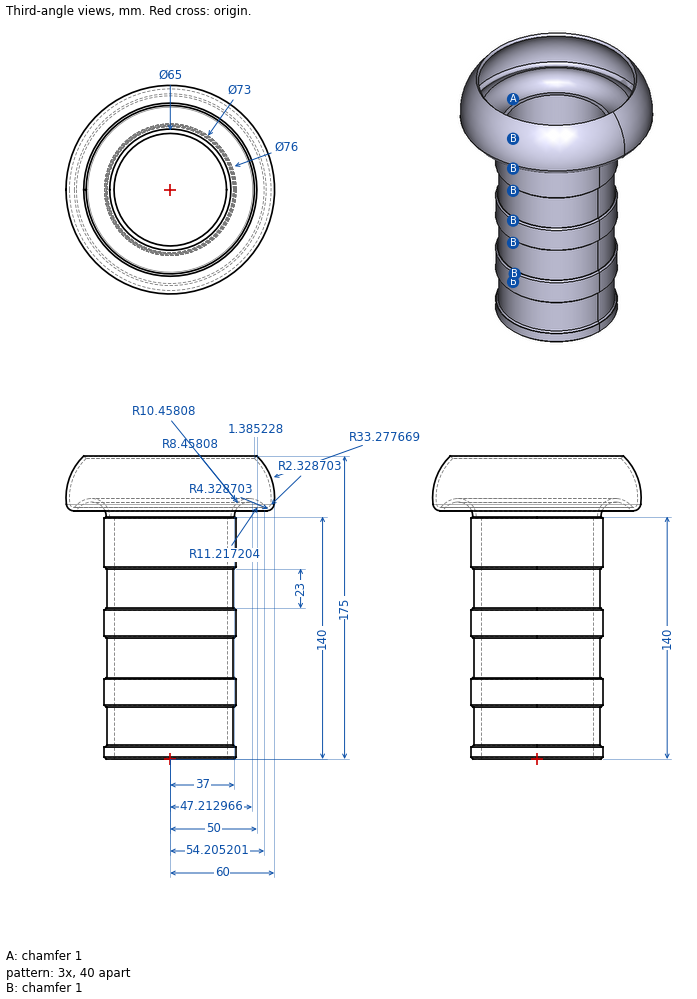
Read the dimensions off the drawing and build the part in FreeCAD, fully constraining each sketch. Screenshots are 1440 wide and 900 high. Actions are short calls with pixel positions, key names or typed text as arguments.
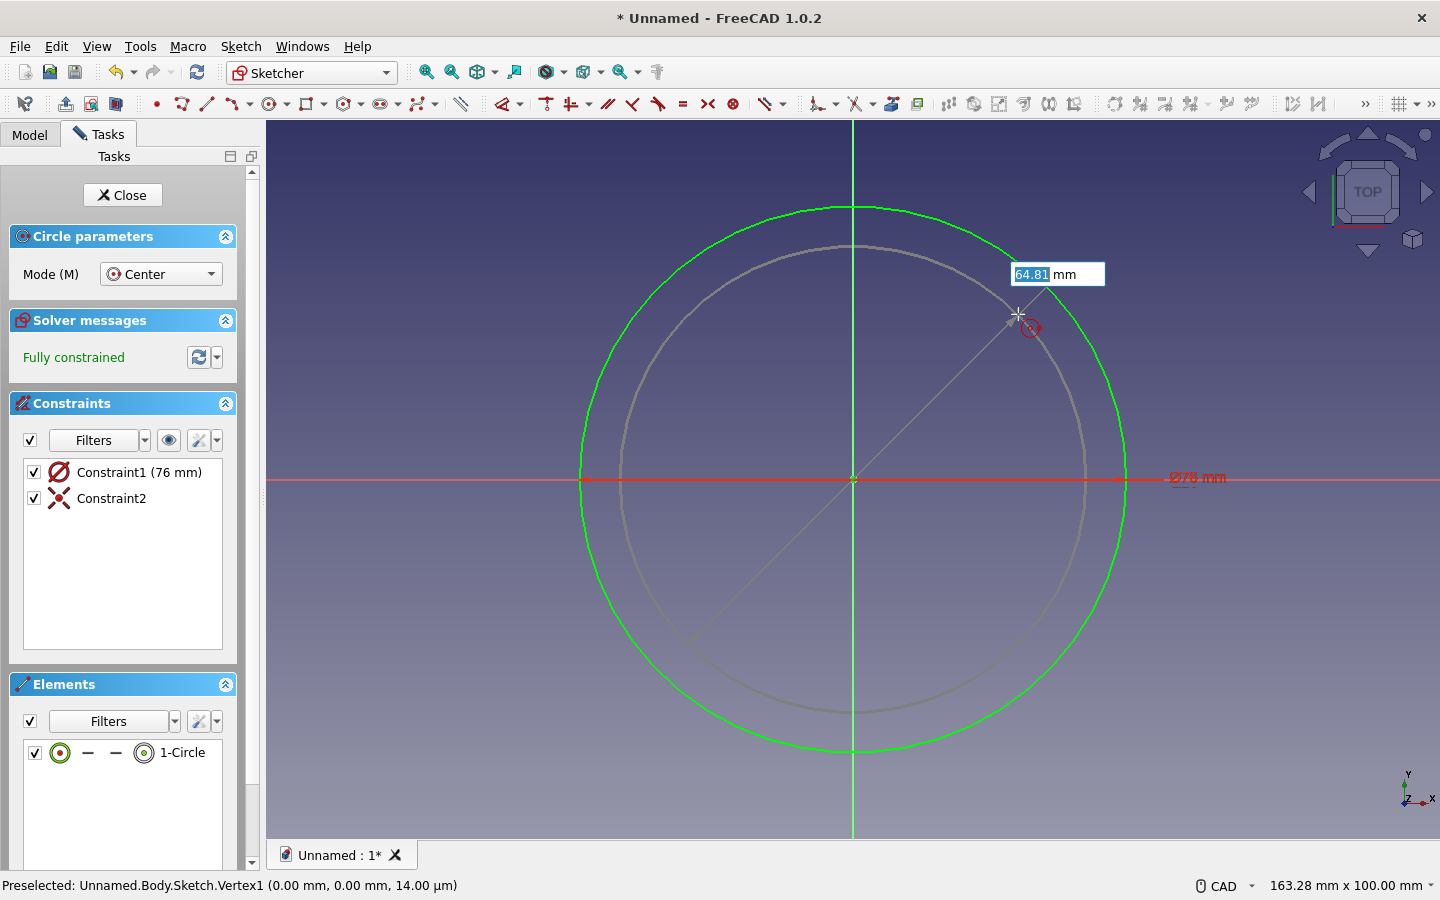
text(65)
key(Return)
key(Escape)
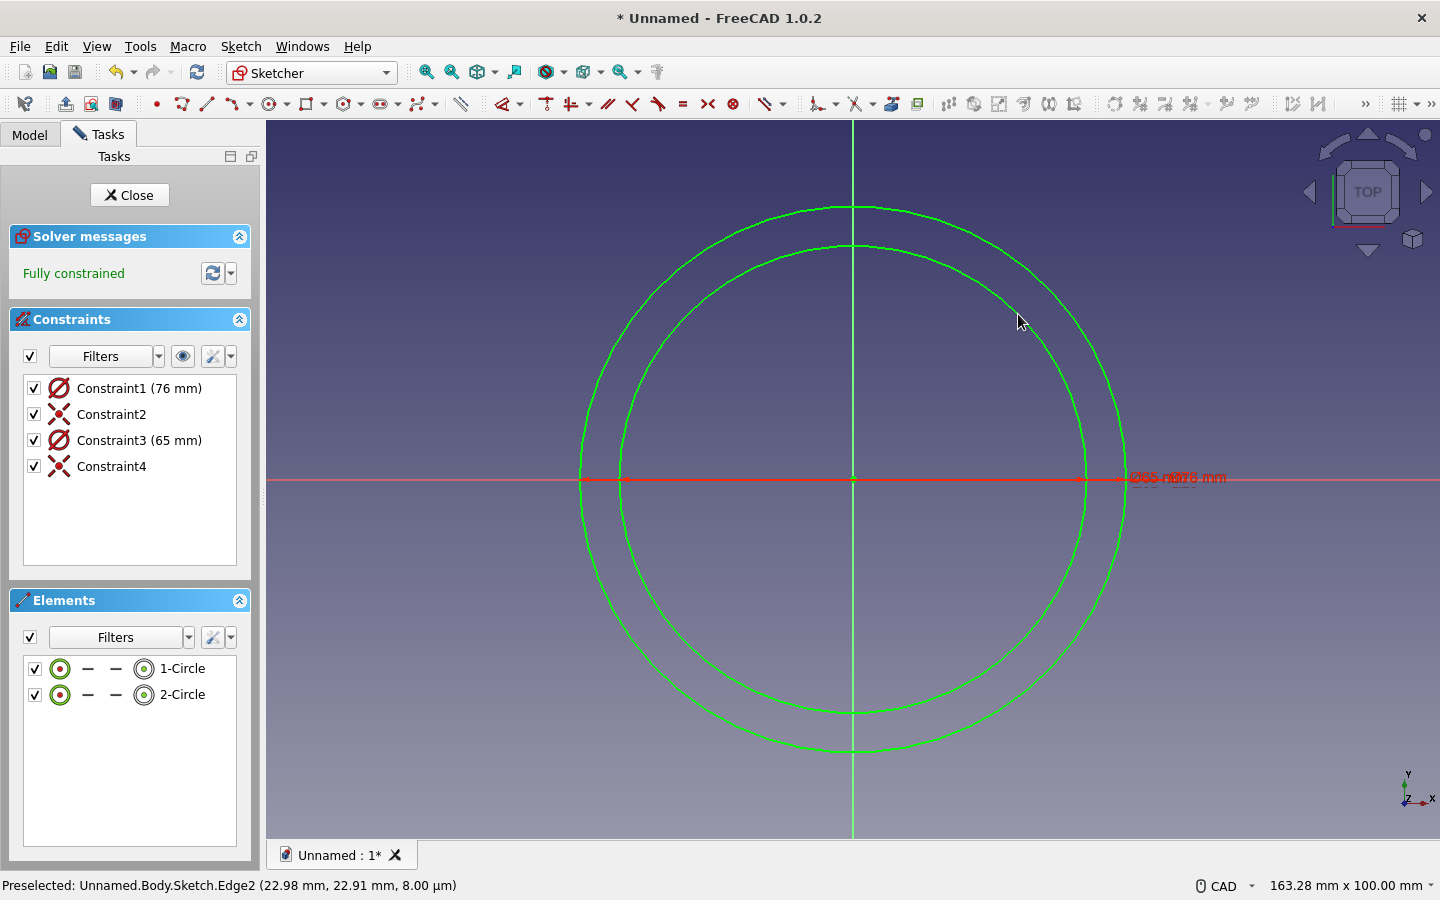
click(130, 195)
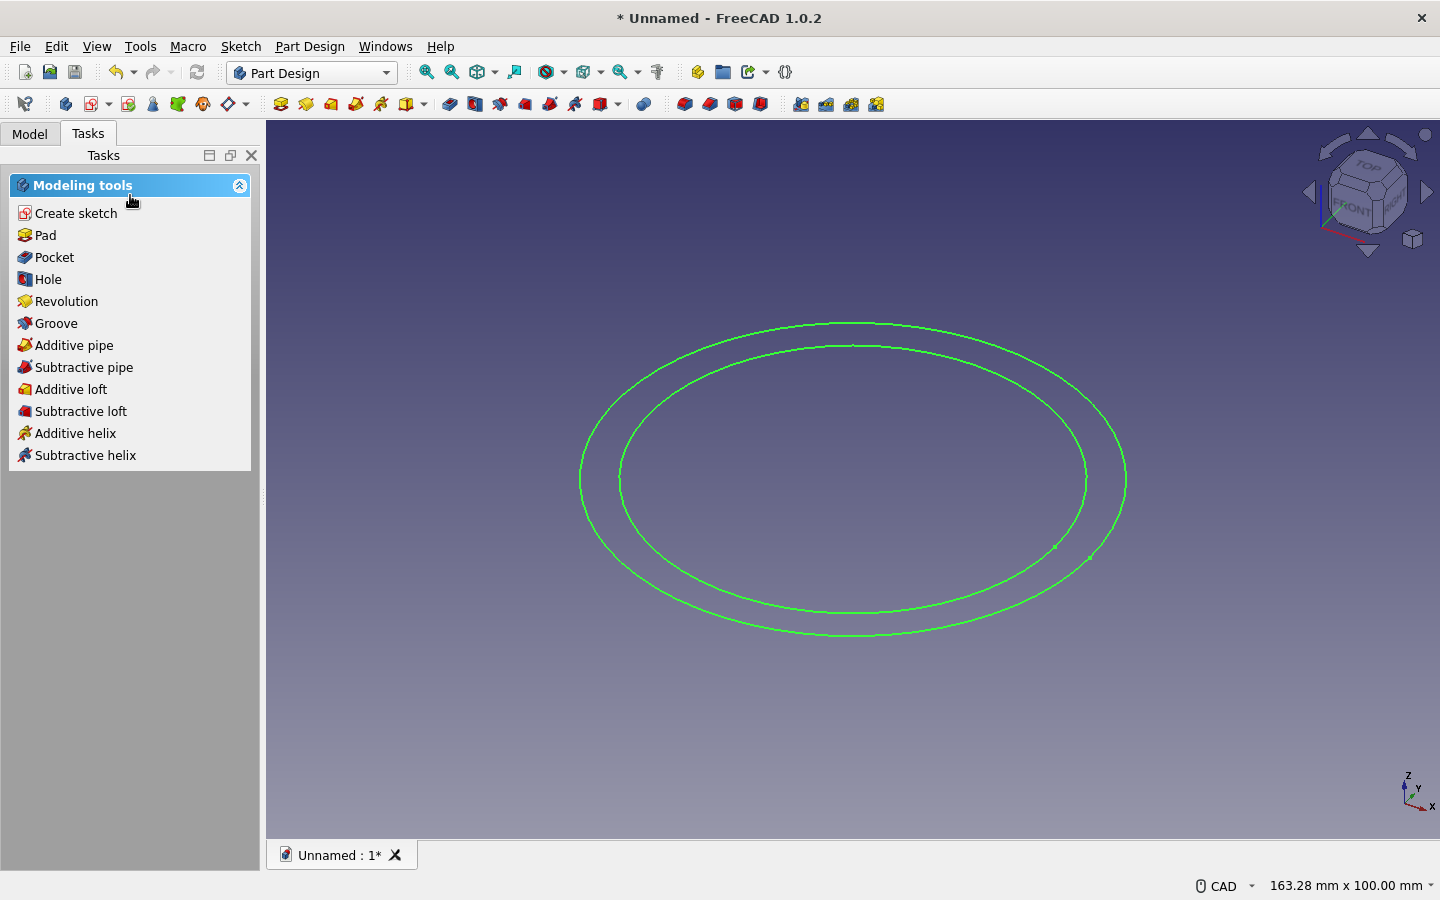
click(281, 104)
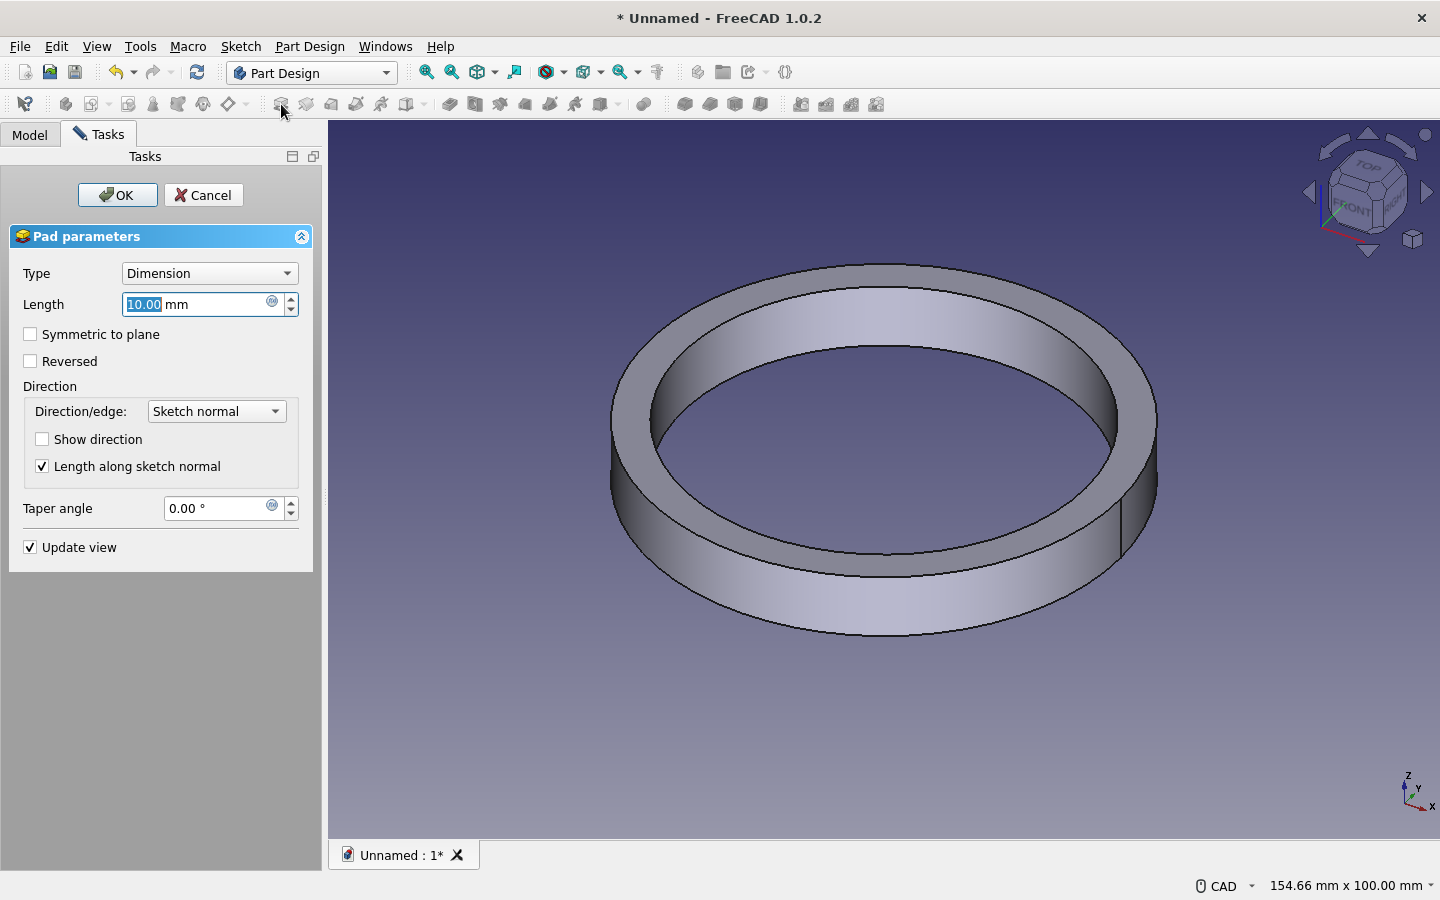
text(140)
key(Tab)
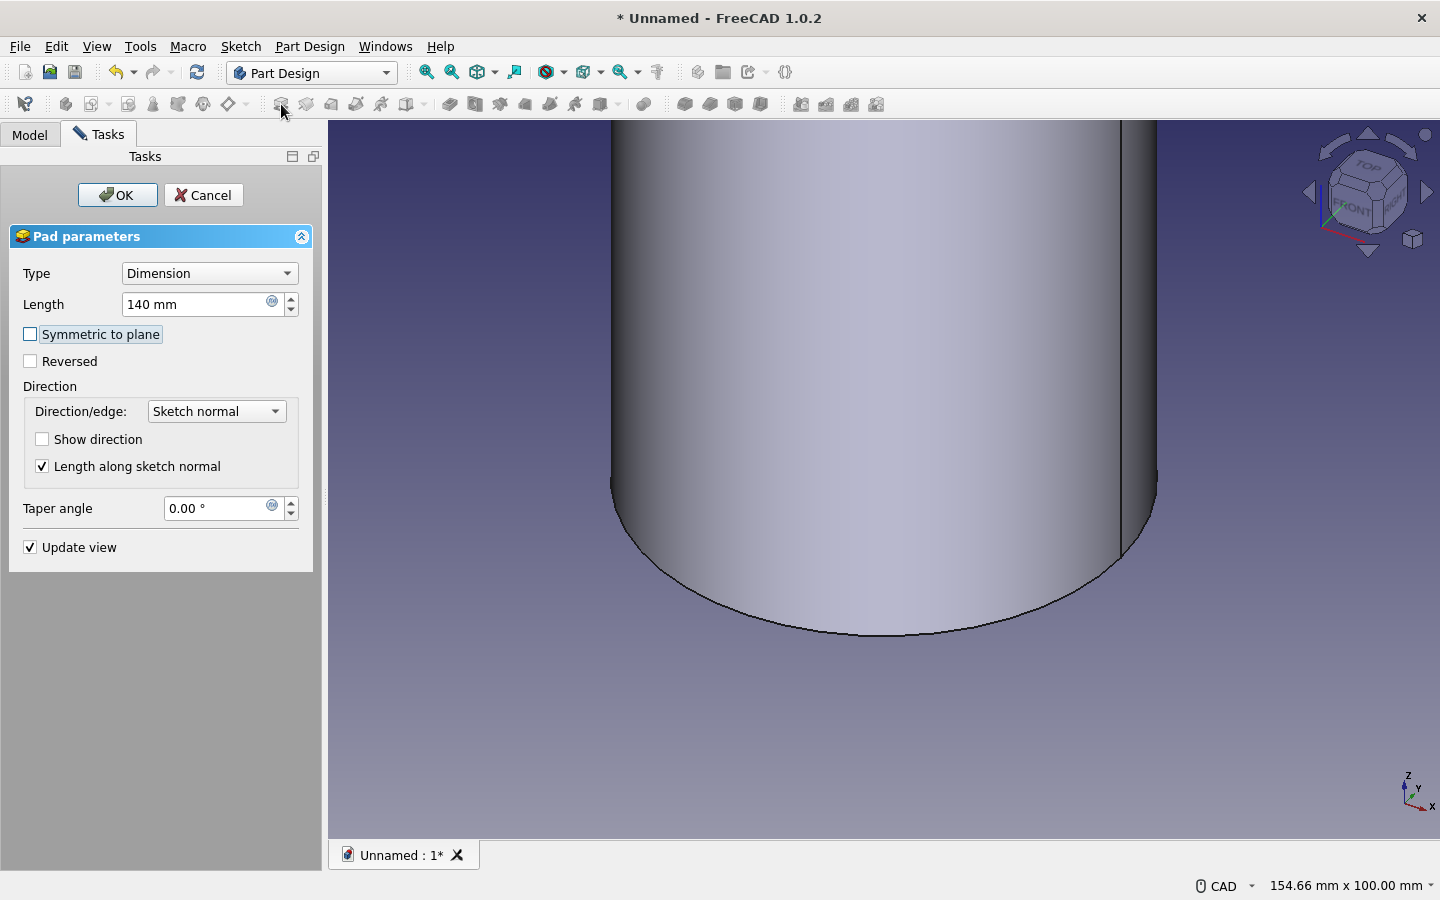
click(118, 195)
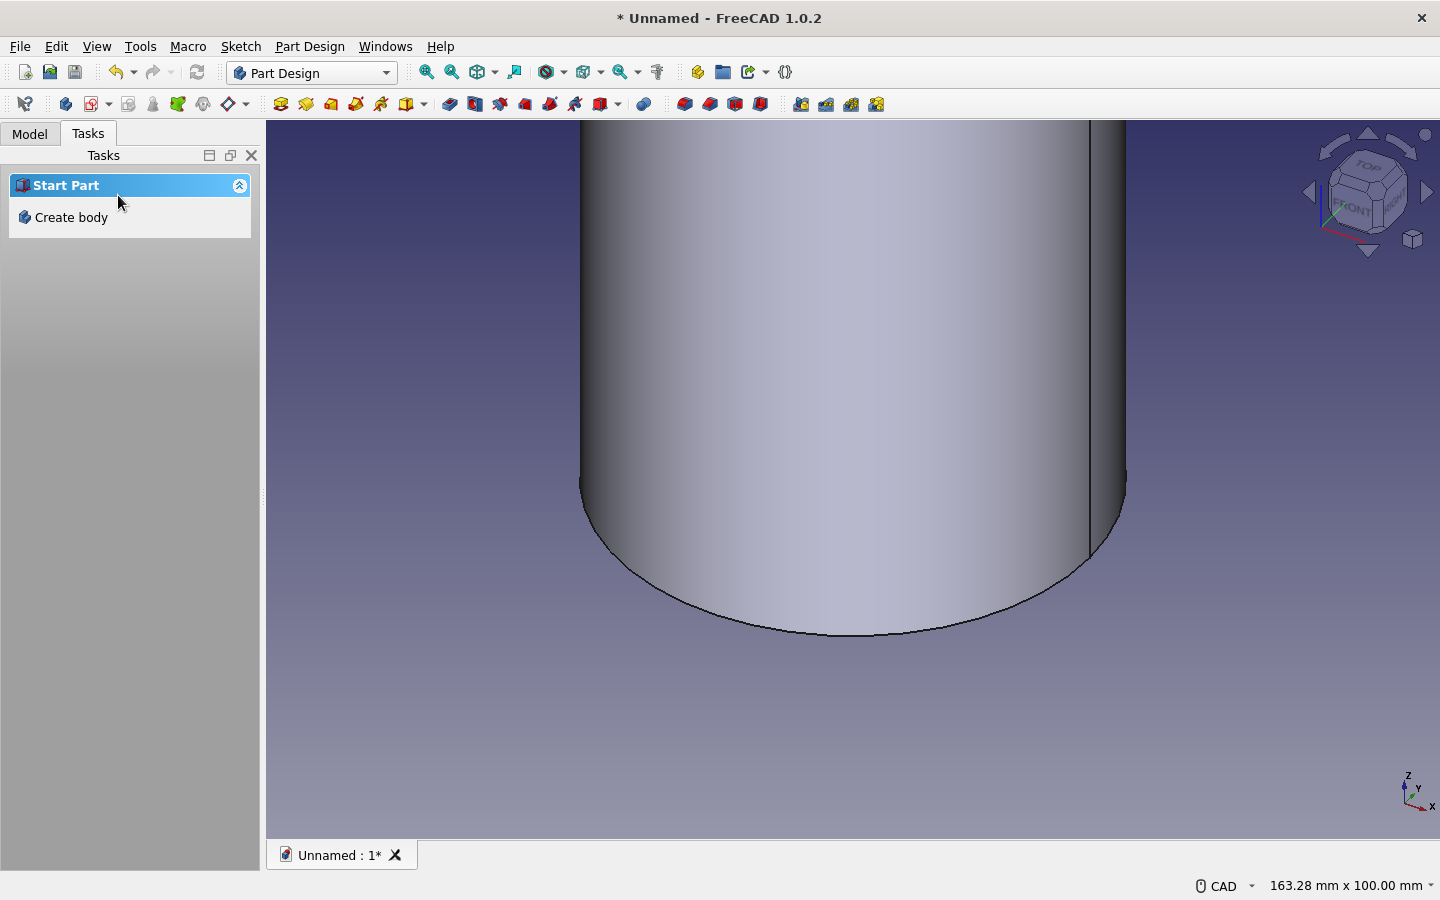
click(427, 72)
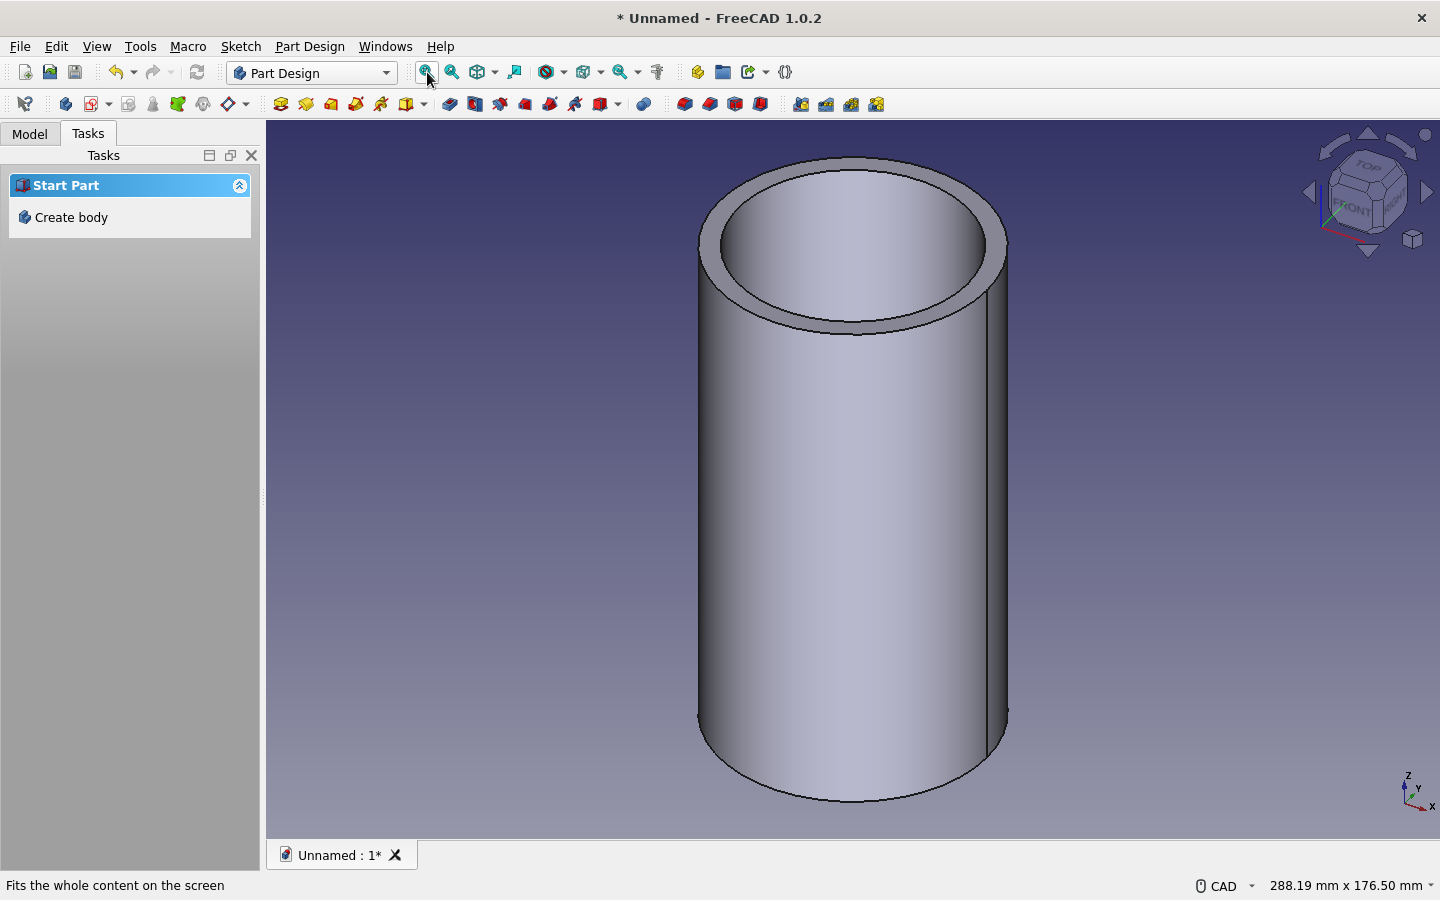
click(699, 254)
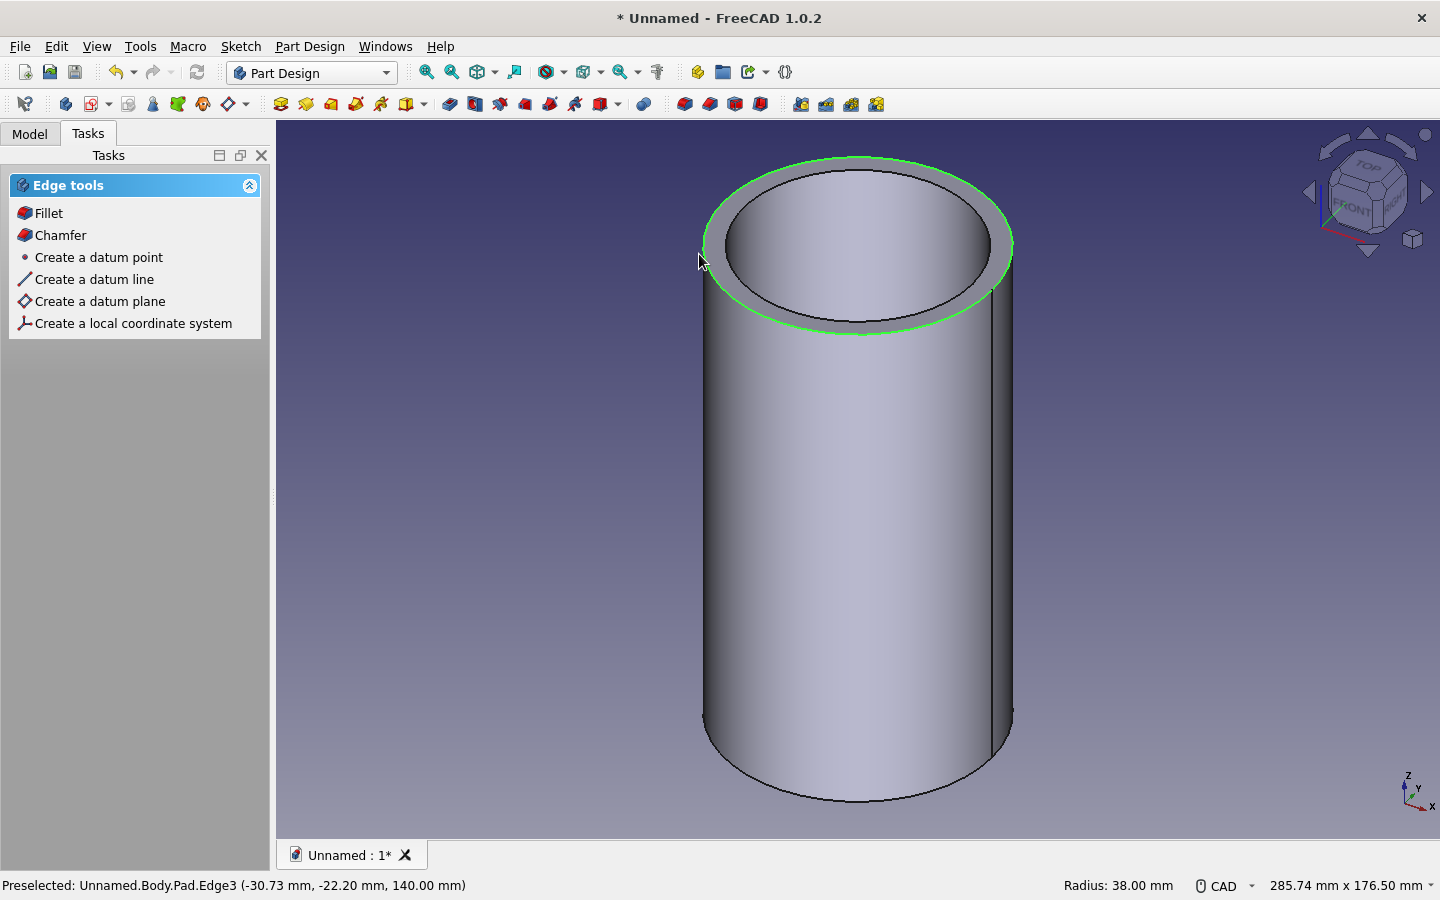
click(710, 104)